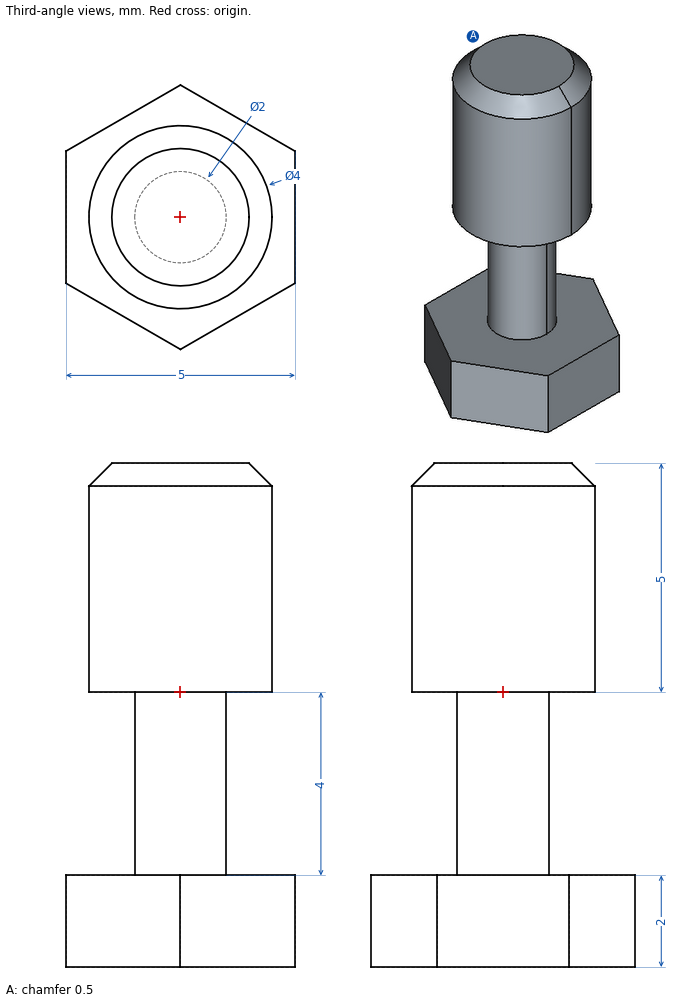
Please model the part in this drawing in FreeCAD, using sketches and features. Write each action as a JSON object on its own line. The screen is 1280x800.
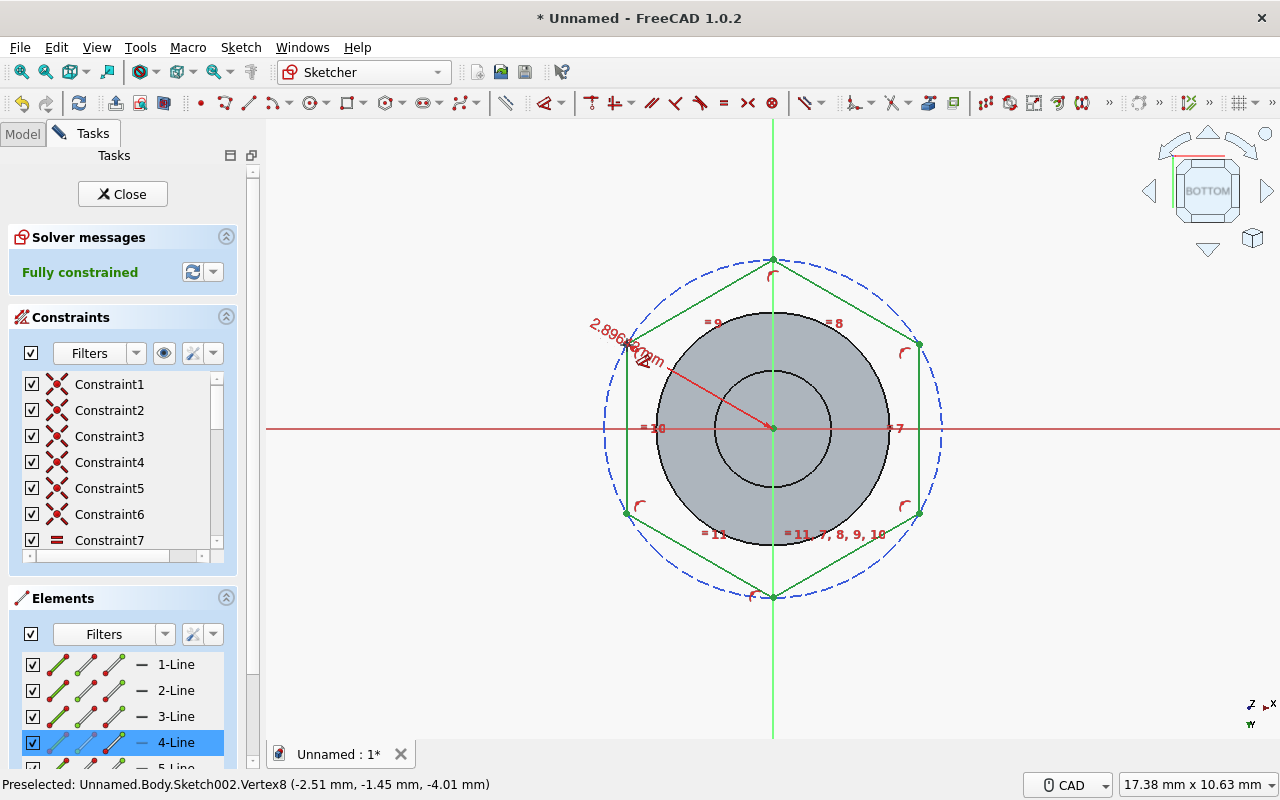
{"action": "left_click", "coordinate": [919, 513]}
{"action": "left_click", "coordinate": [671, 595]}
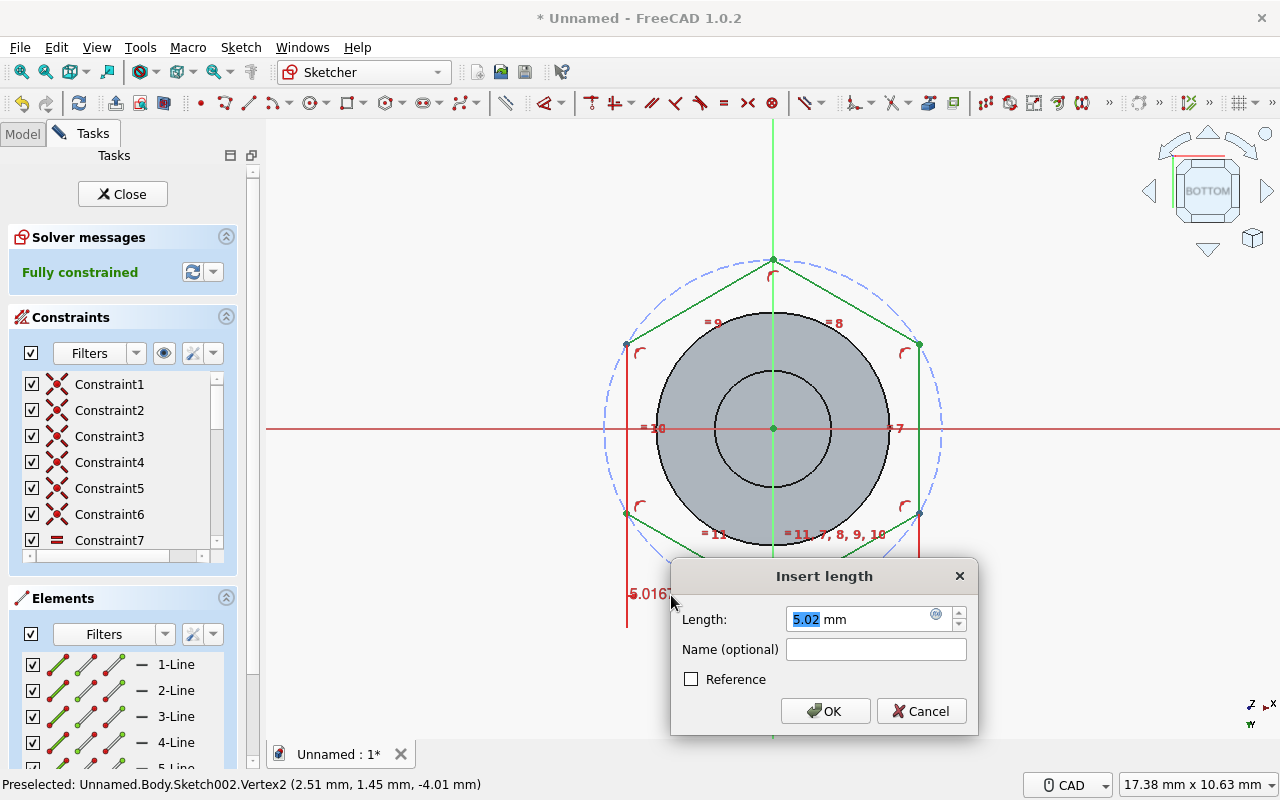
{"action": "type", "text": "5"}
{"action": "key", "text": "Return"}
{"action": "key", "text": "Escape"}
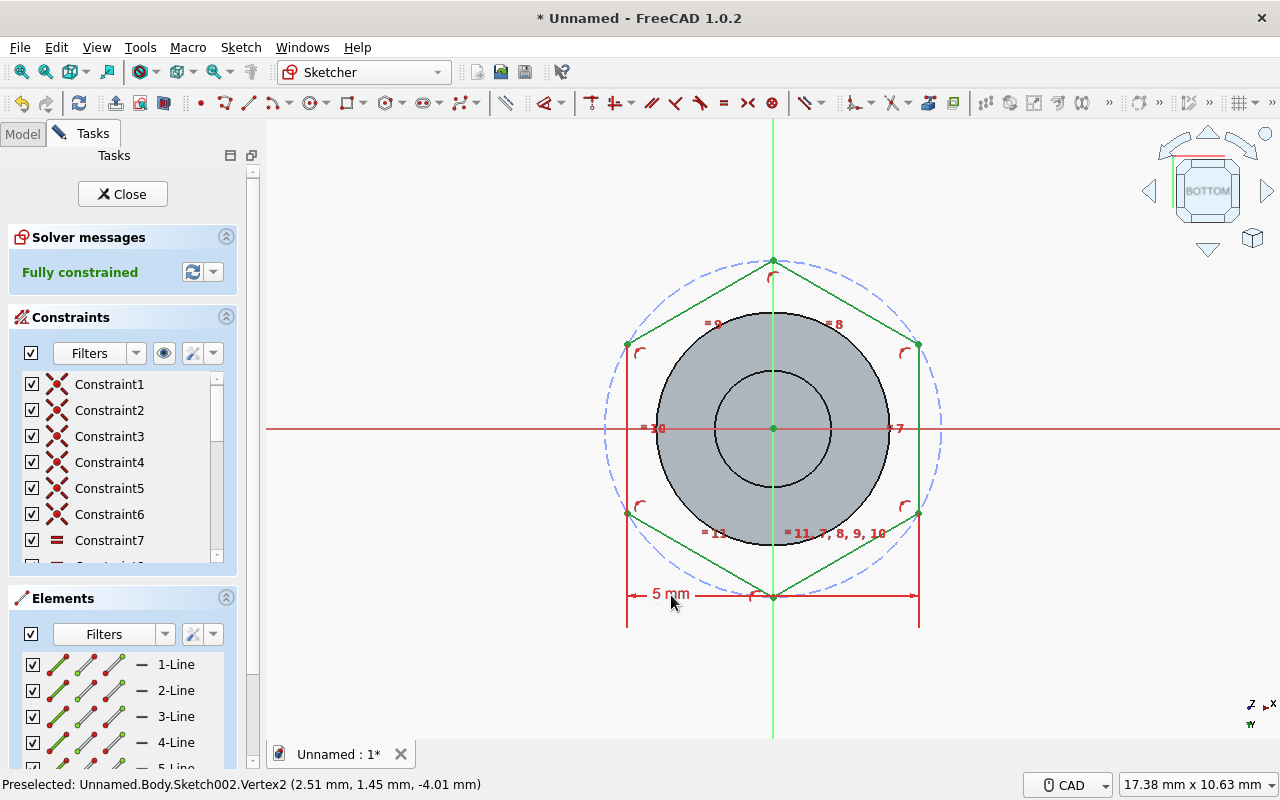
{"action": "left_click", "coordinate": [123, 194]}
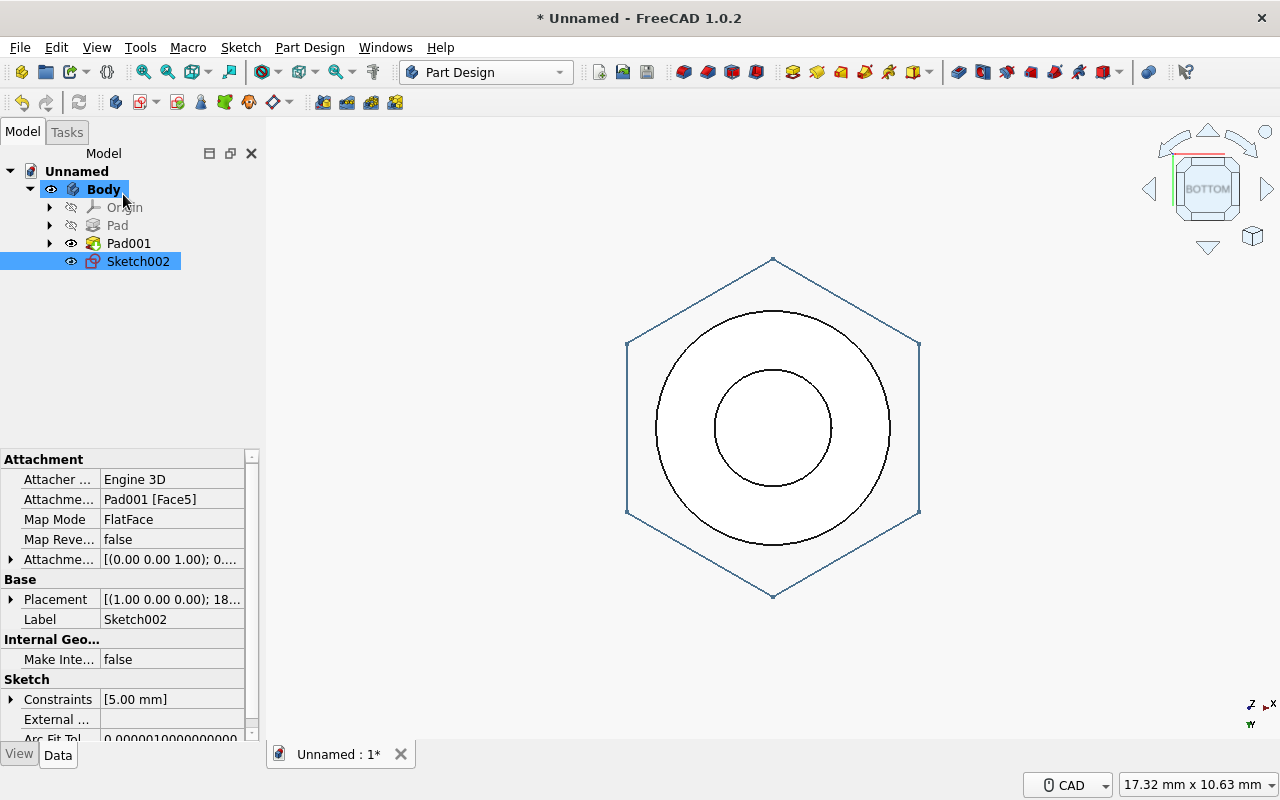
{"action": "left_click", "coordinate": [794, 72]}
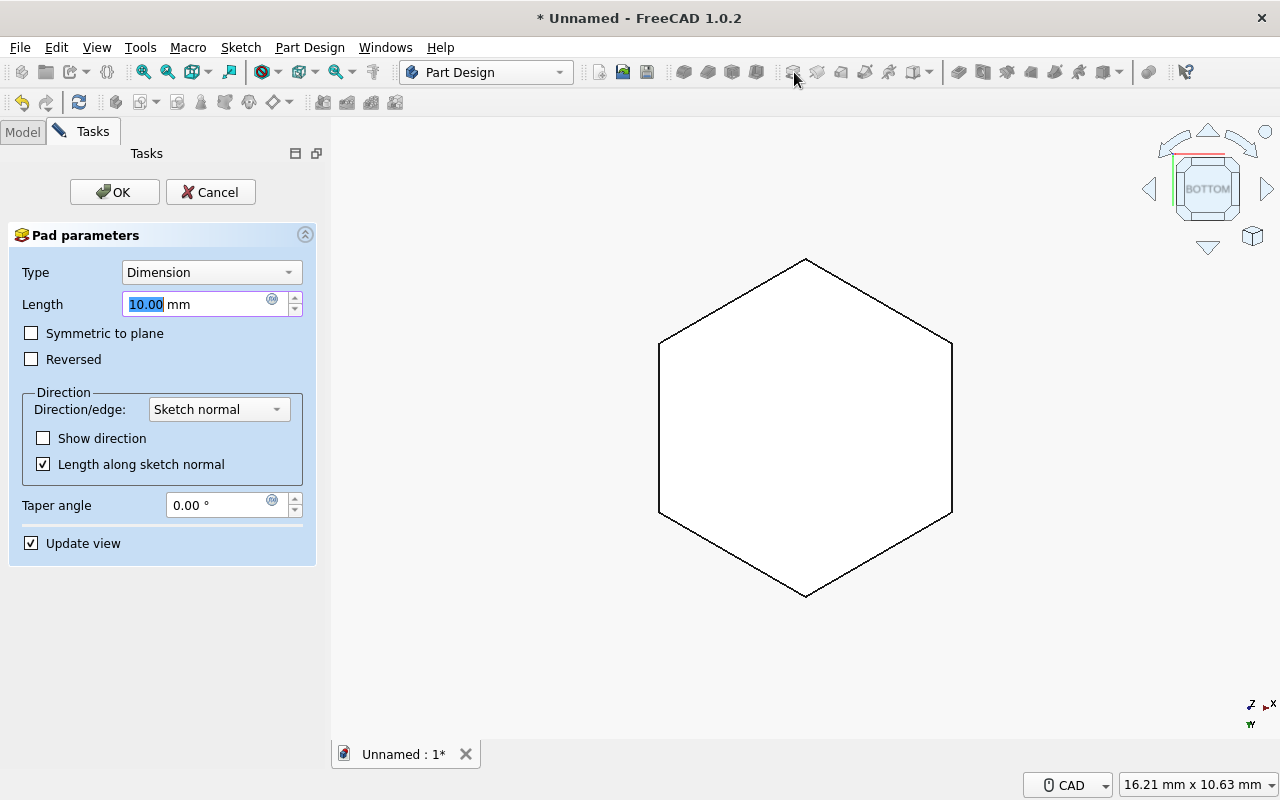
{"action": "type", "text": "2"}
{"action": "key", "text": "Tab"}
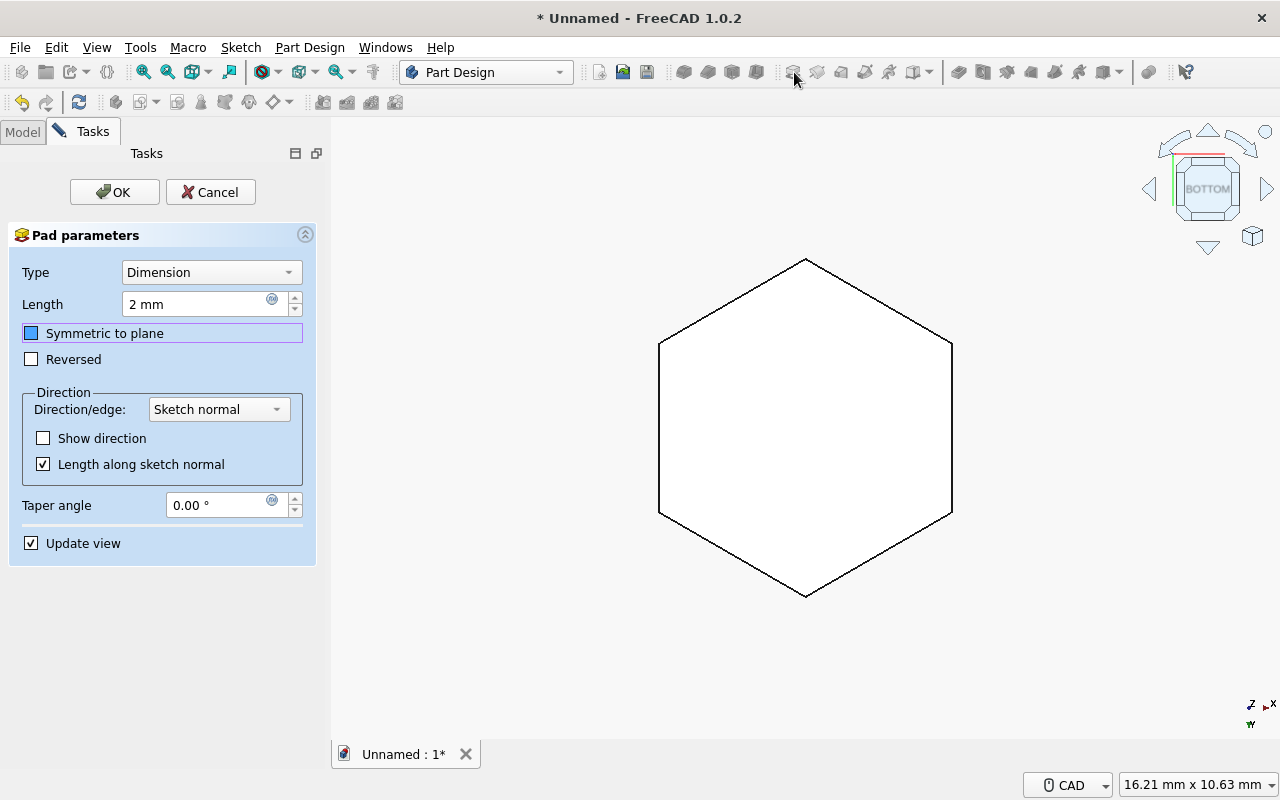
{"action": "left_click", "coordinate": [115, 192]}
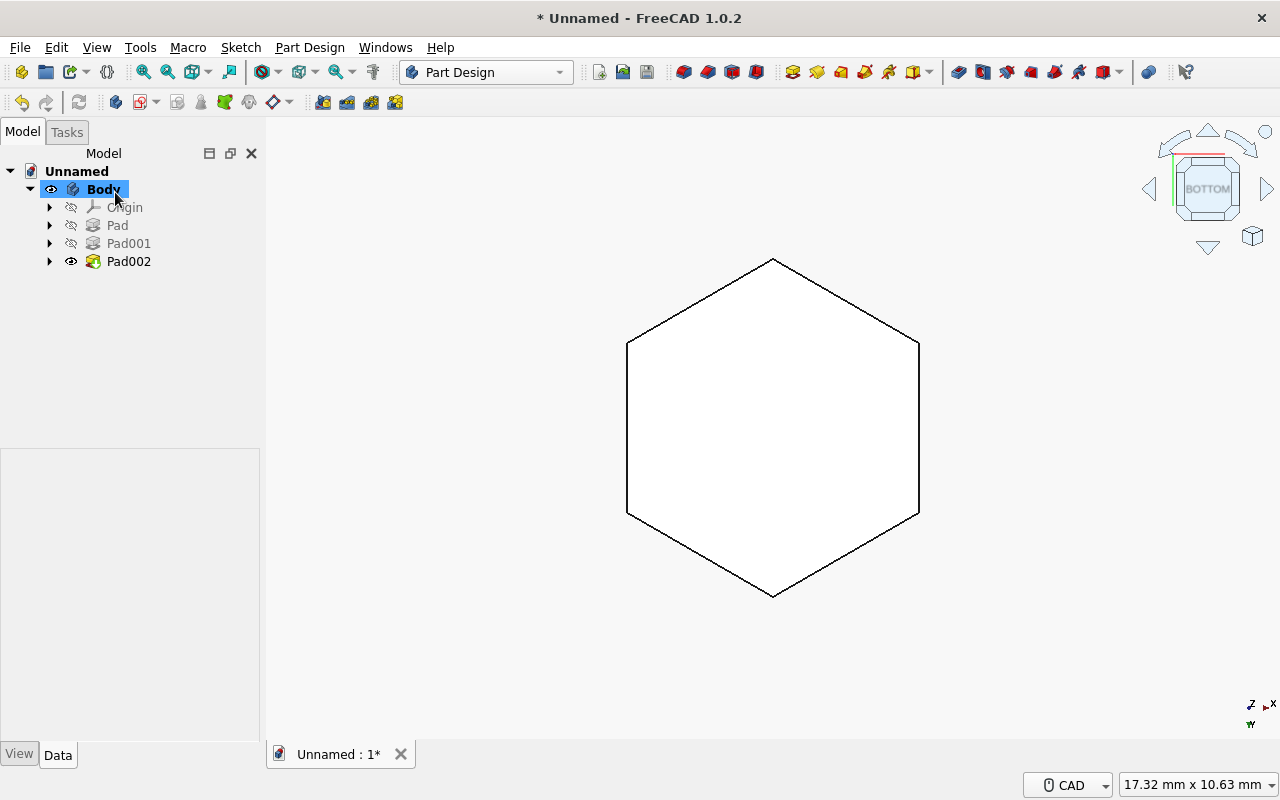
{"action": "key", "text": "0"}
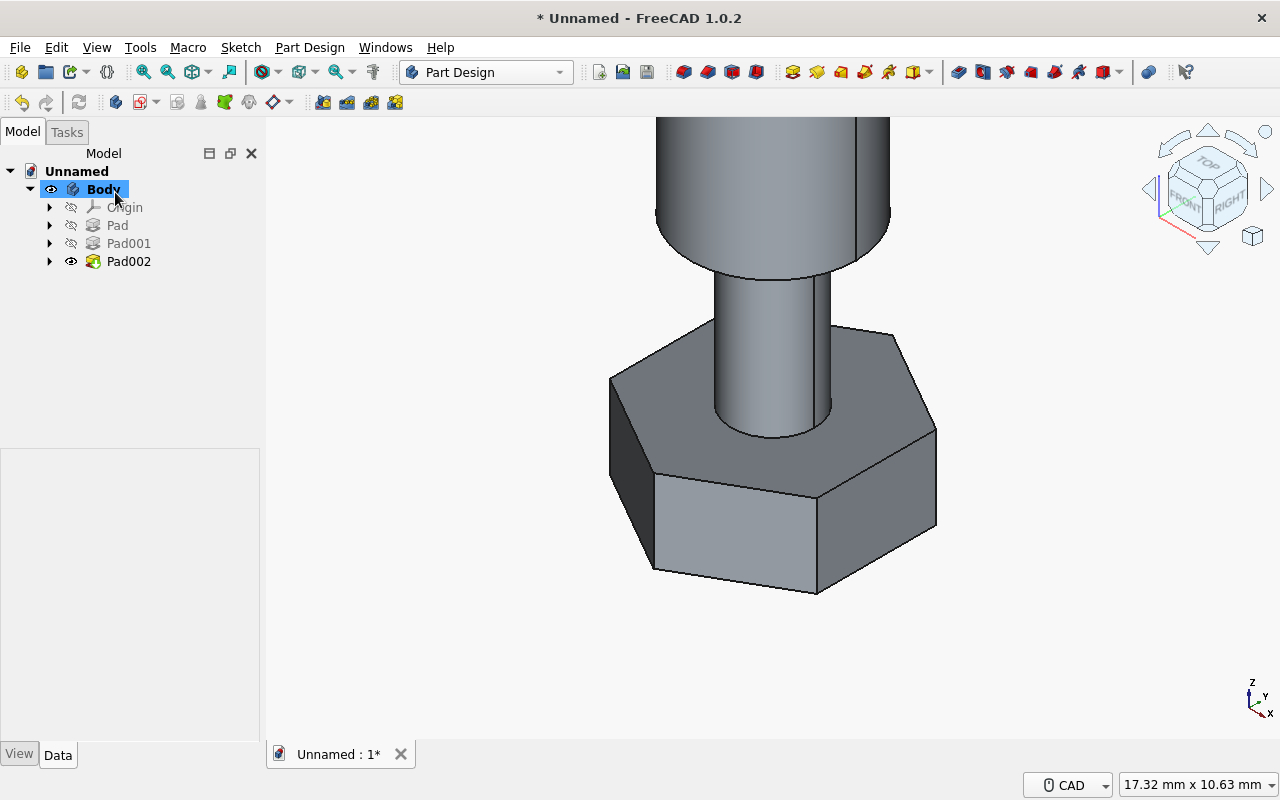
{"action": "left_click", "coordinate": [144, 72]}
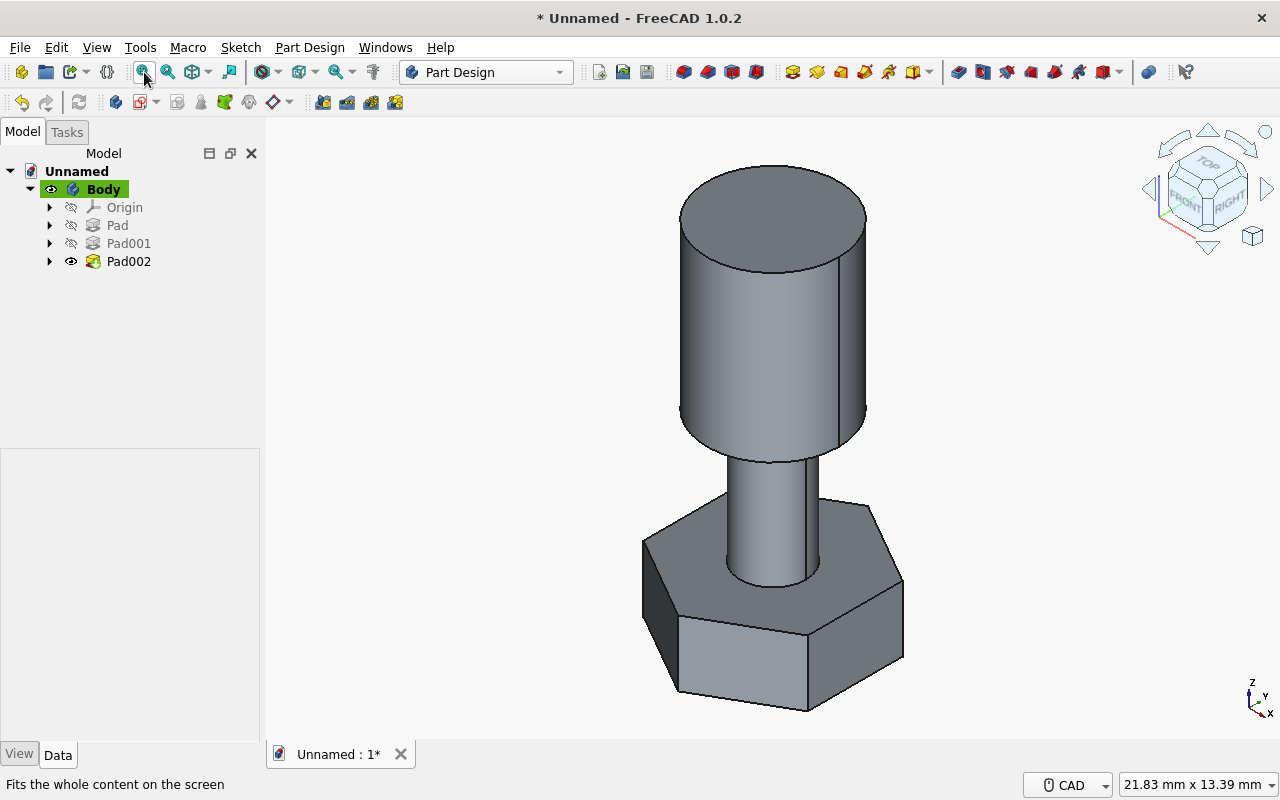
{"action": "left_click", "coordinate": [690, 243]}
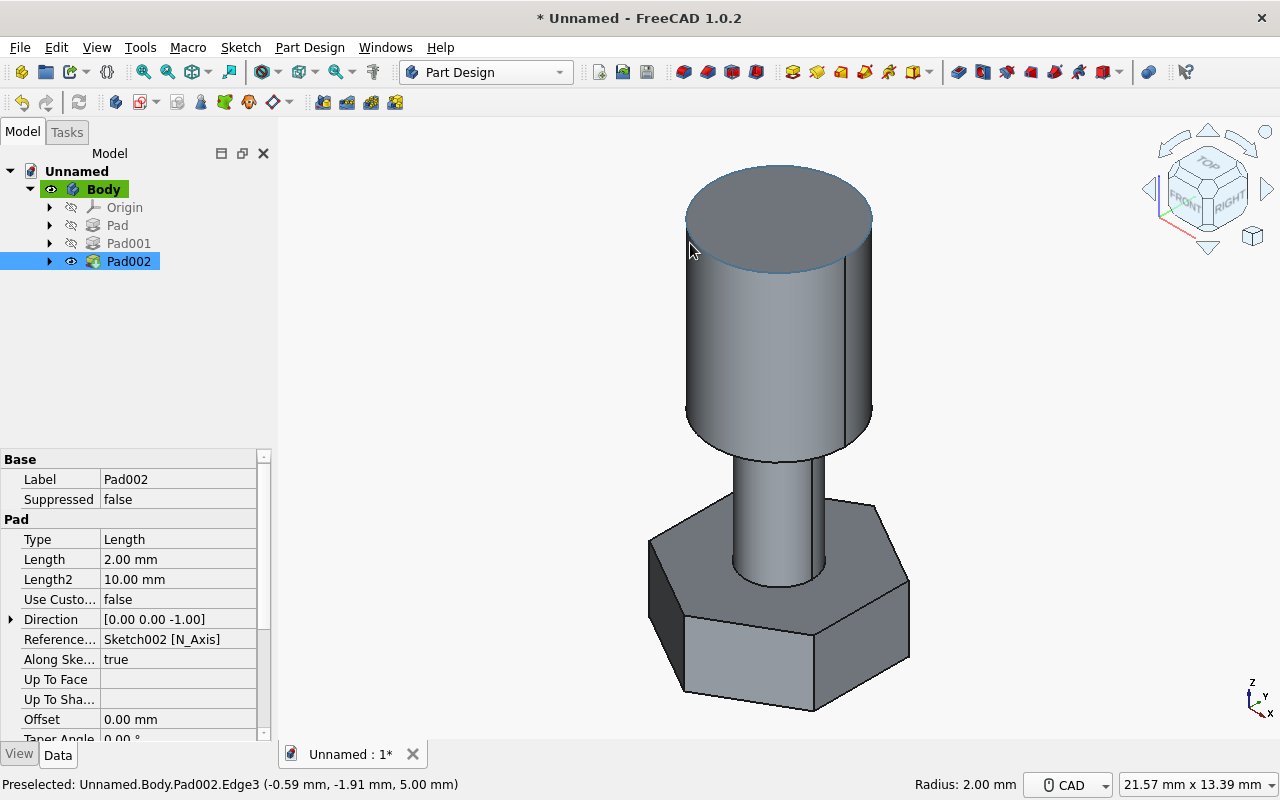
{"action": "left_click", "coordinate": [708, 72]}